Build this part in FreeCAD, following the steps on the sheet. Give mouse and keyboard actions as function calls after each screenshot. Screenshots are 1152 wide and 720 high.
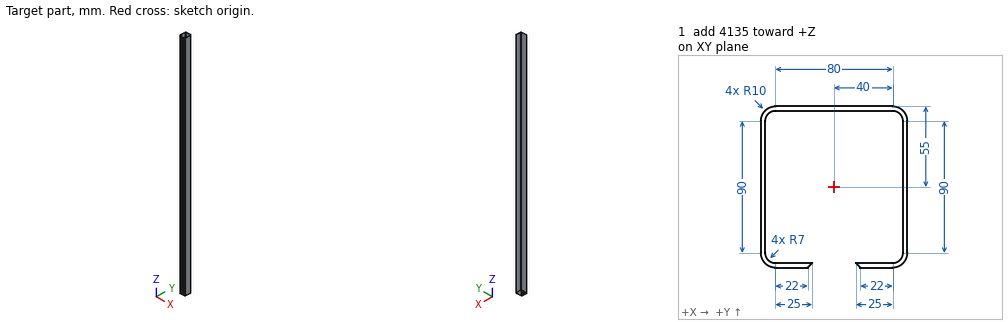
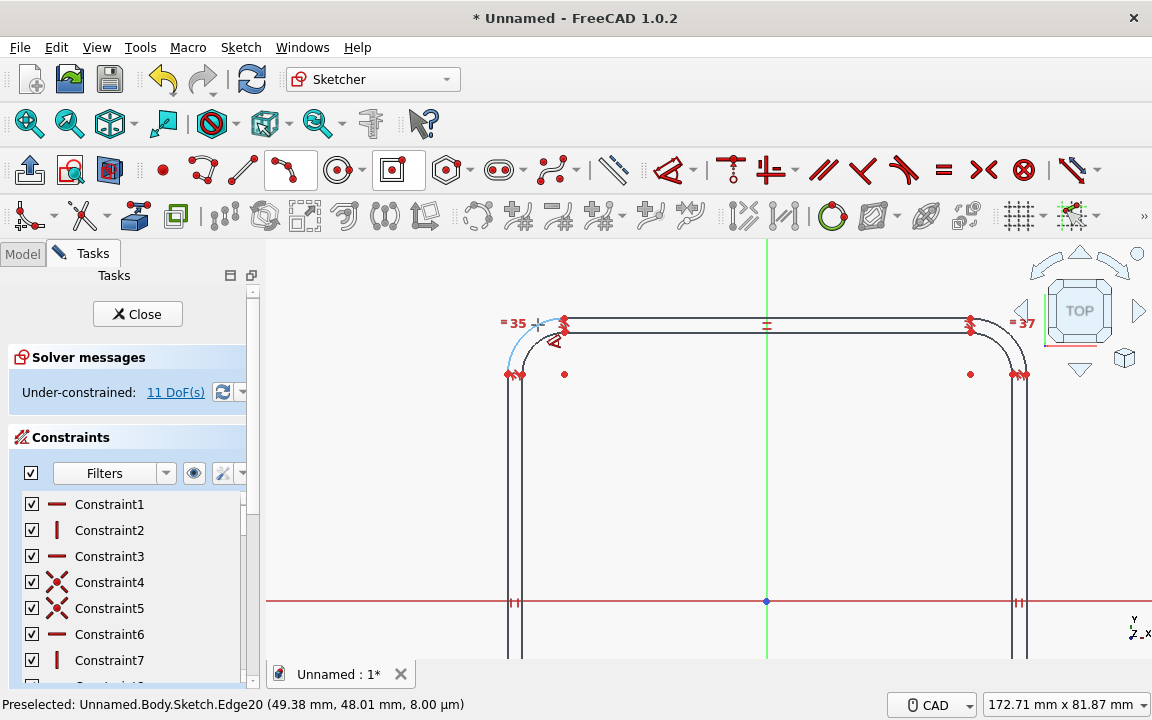
click(539, 325)
click(525, 296)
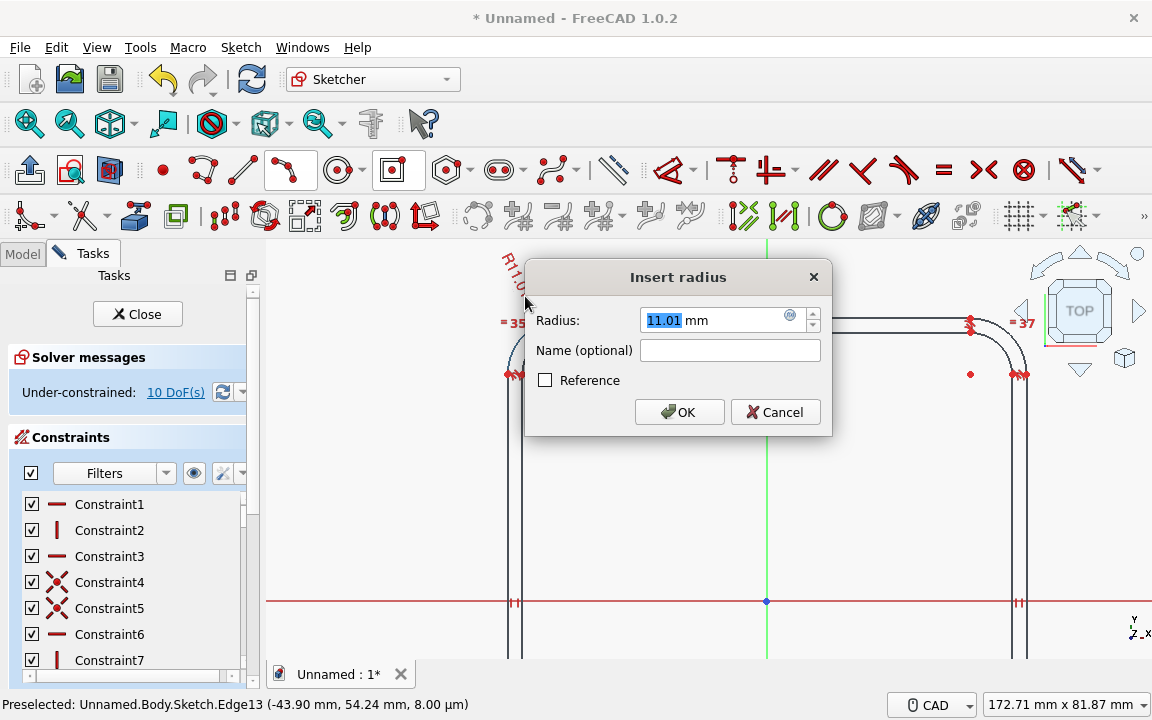
text(10)
key(Return)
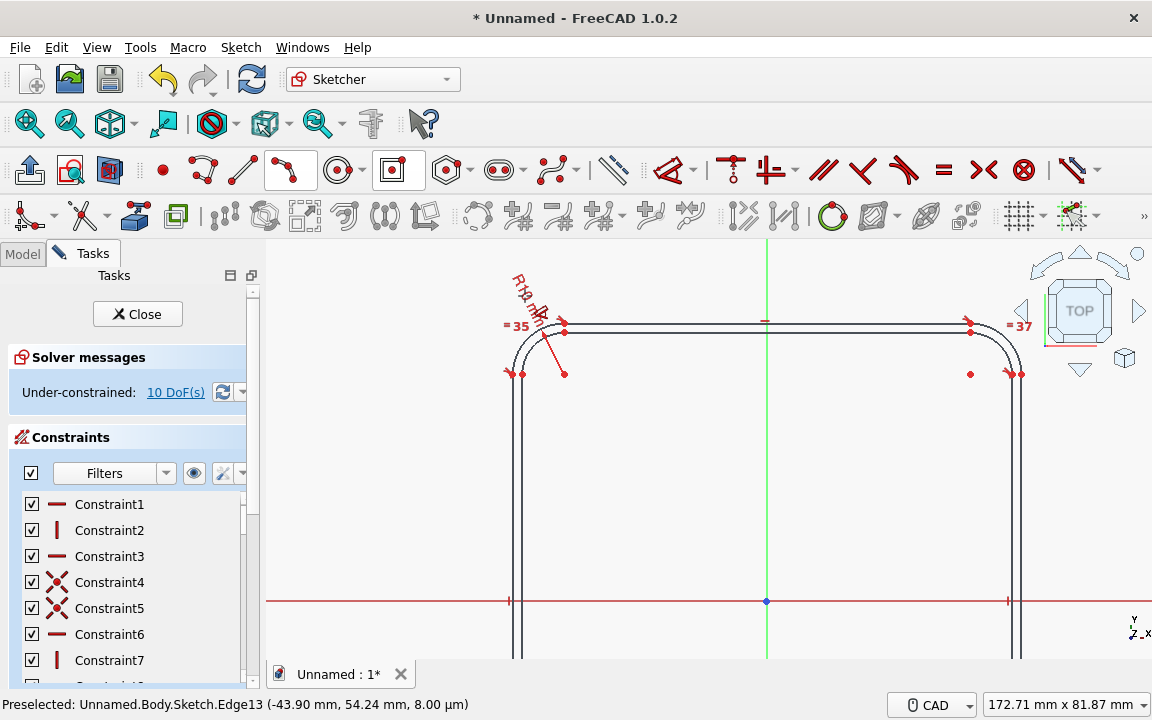
scroll(537, 325, down, 4)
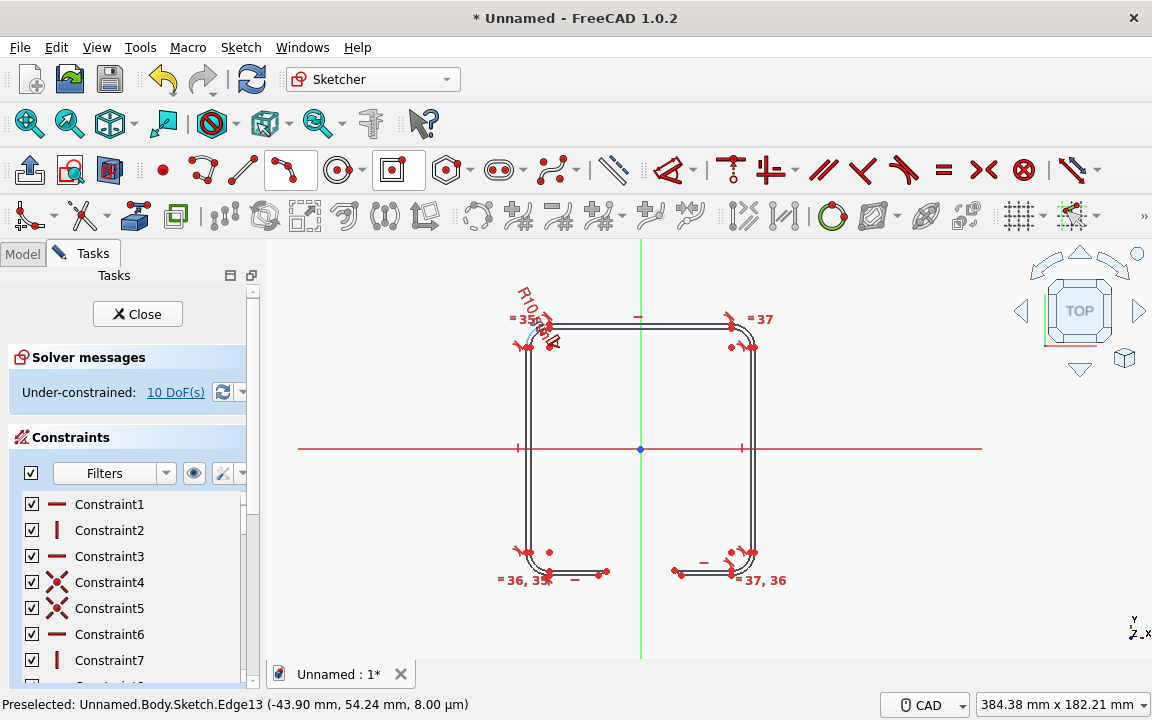
scroll(533, 561, up, 6)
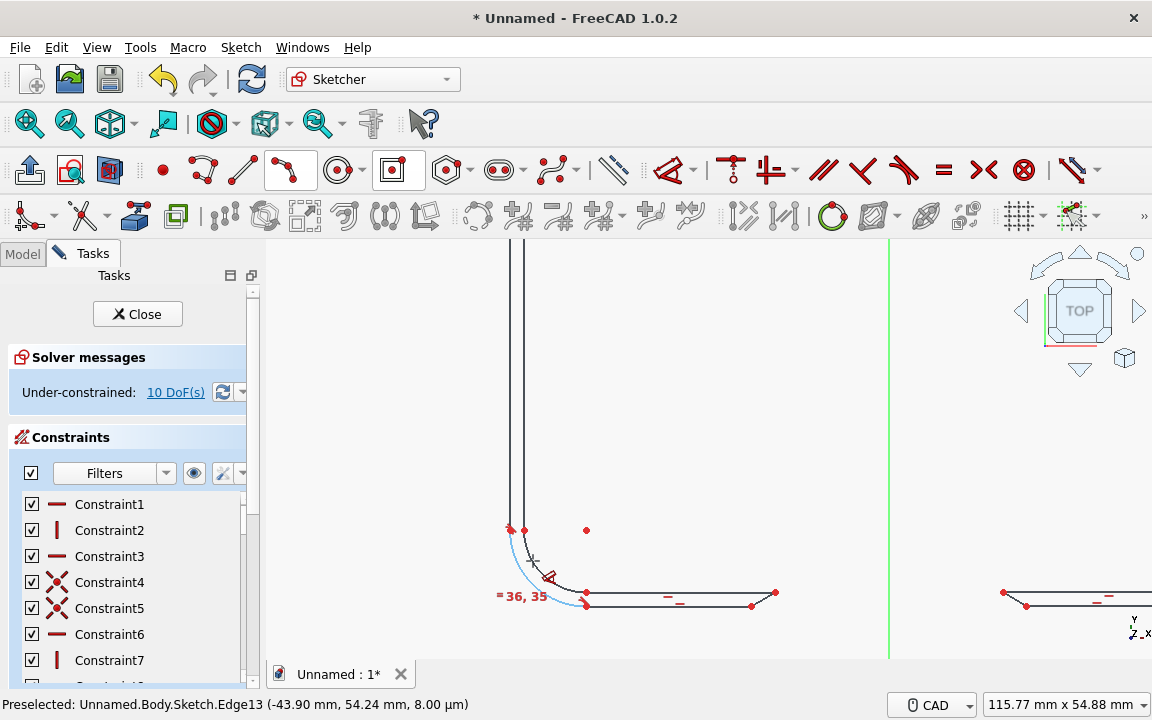
click(531, 558)
click(502, 572)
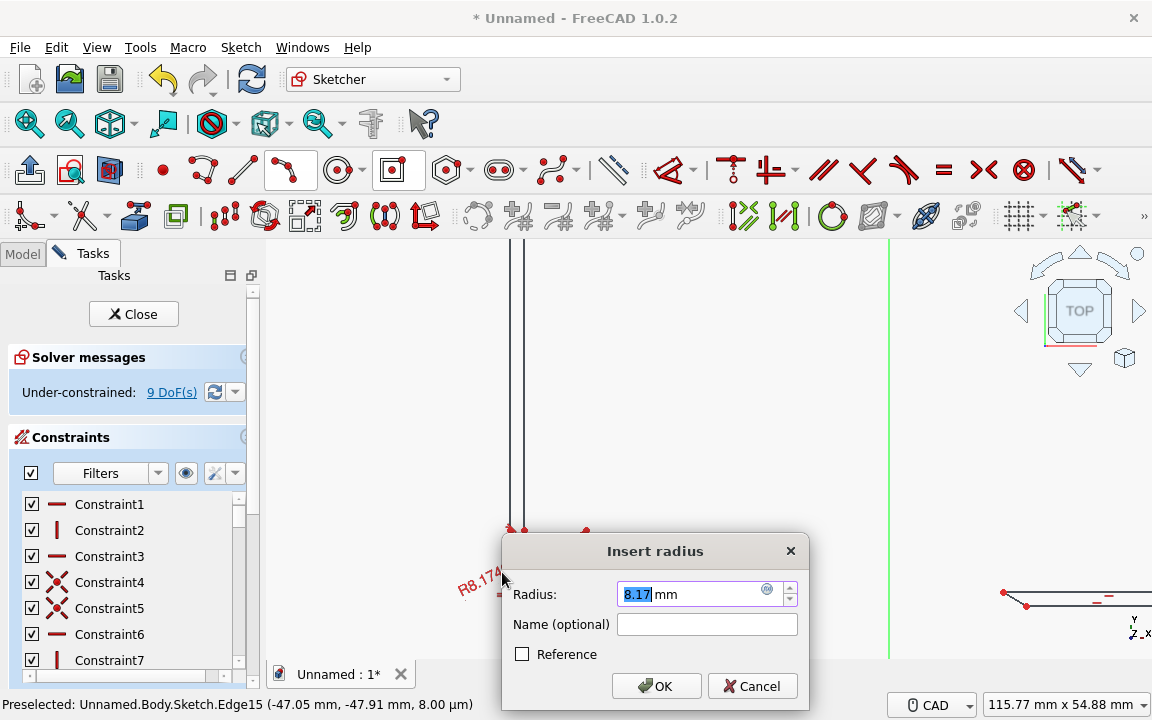
text(7)
key(Return)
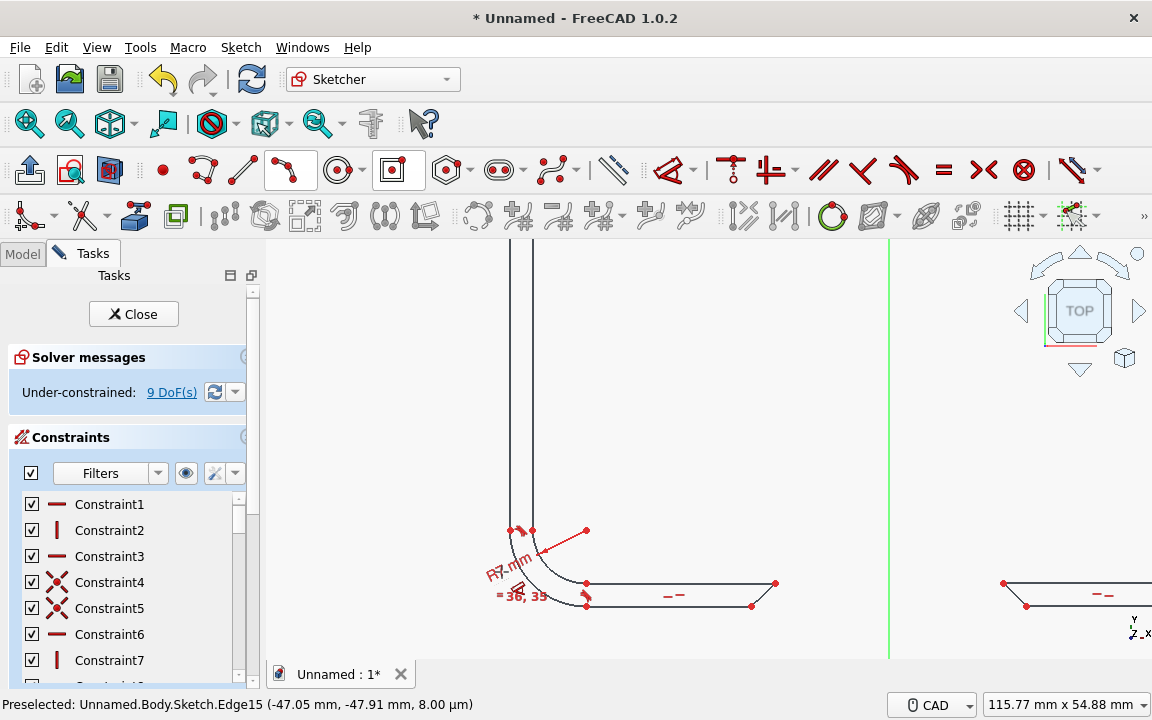
scroll(533, 561, down, 6)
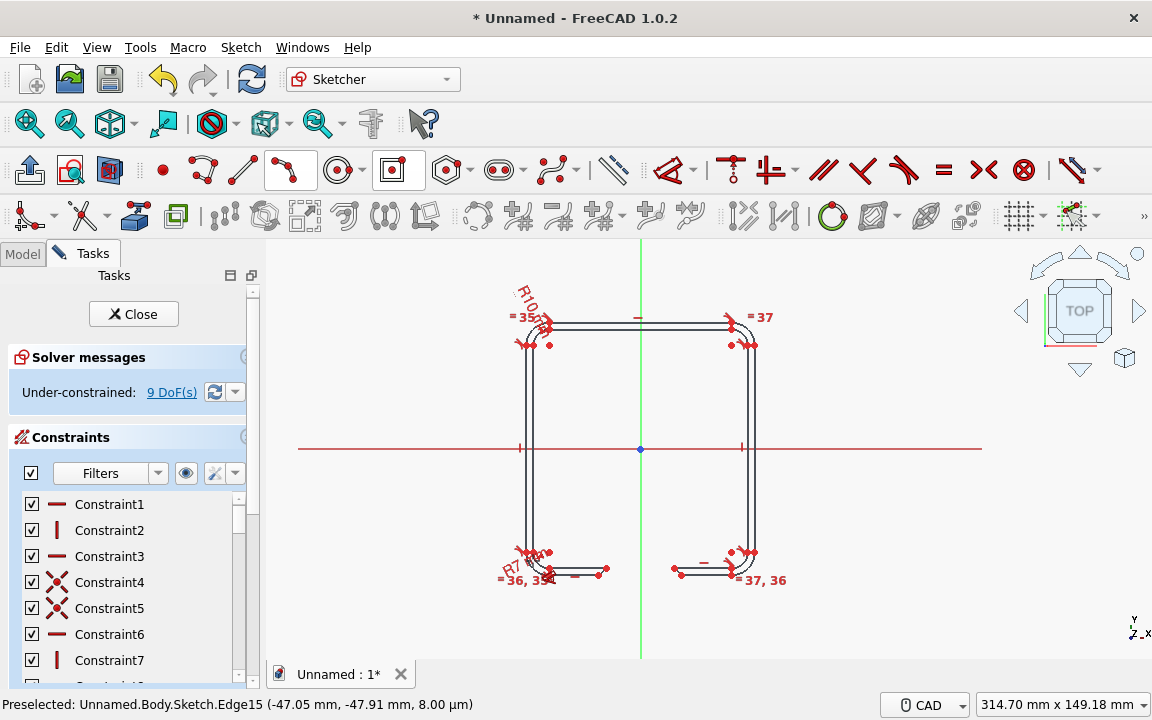
scroll(677, 323, up, 4)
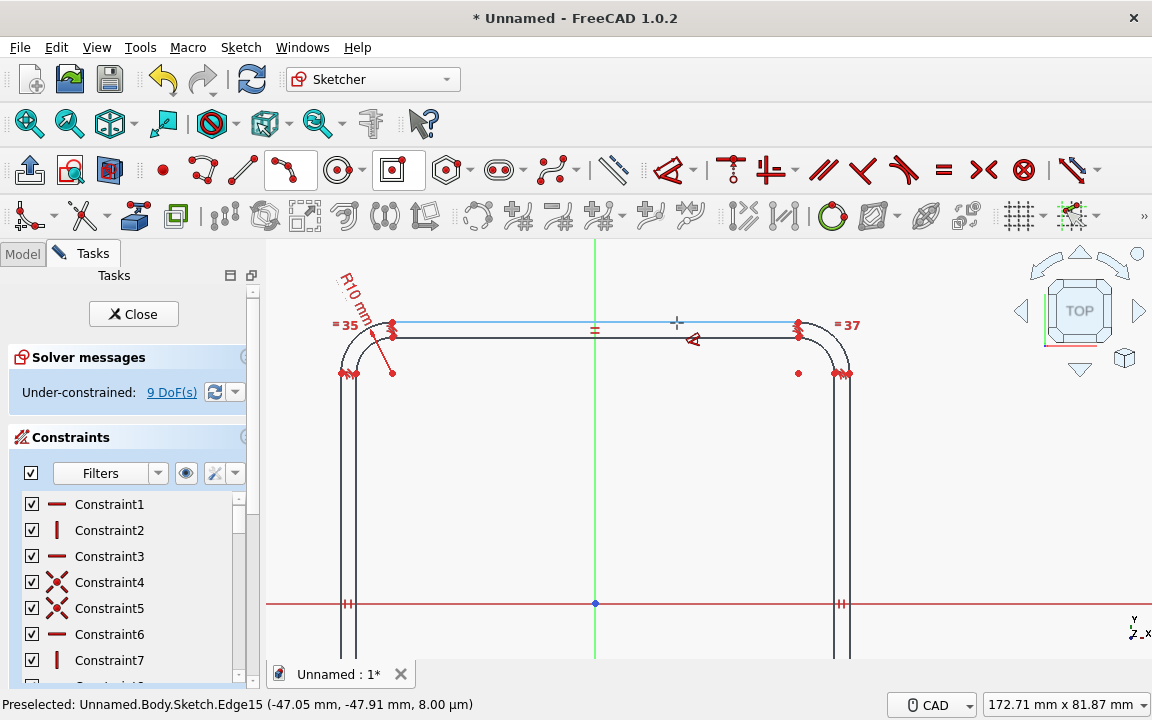
click(677, 322)
click(502, 288)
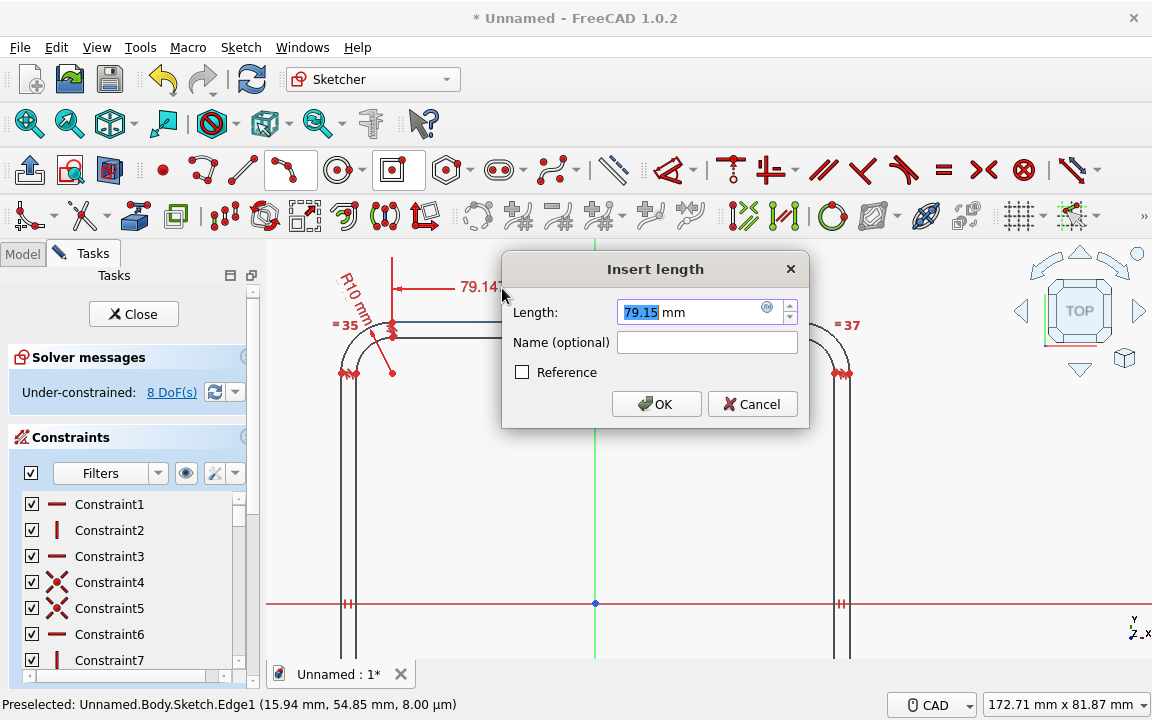
text(80)
key(Return)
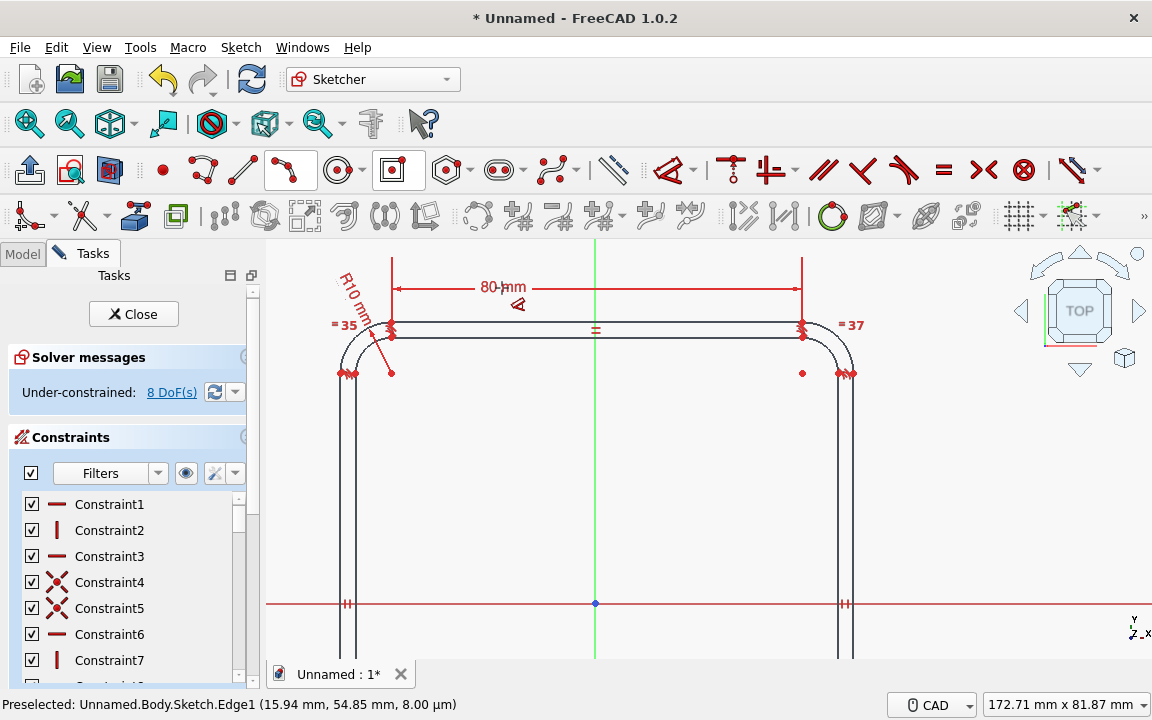
click(340, 511)
click(306, 502)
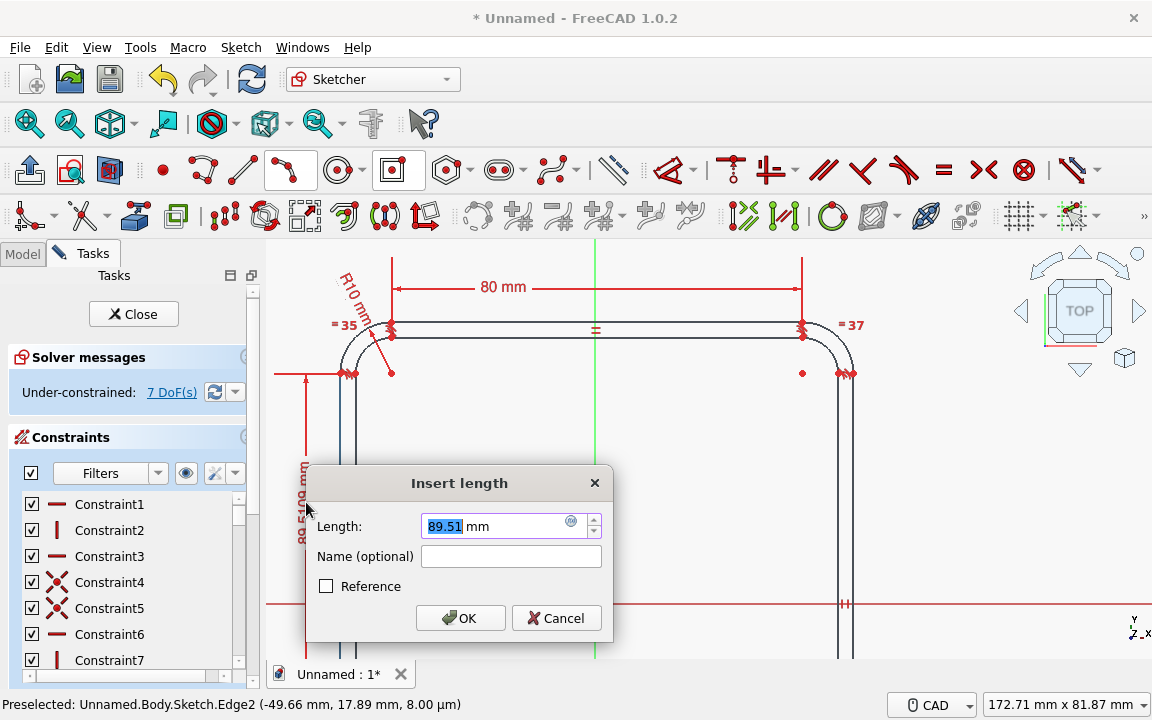
text(90)
key(Return)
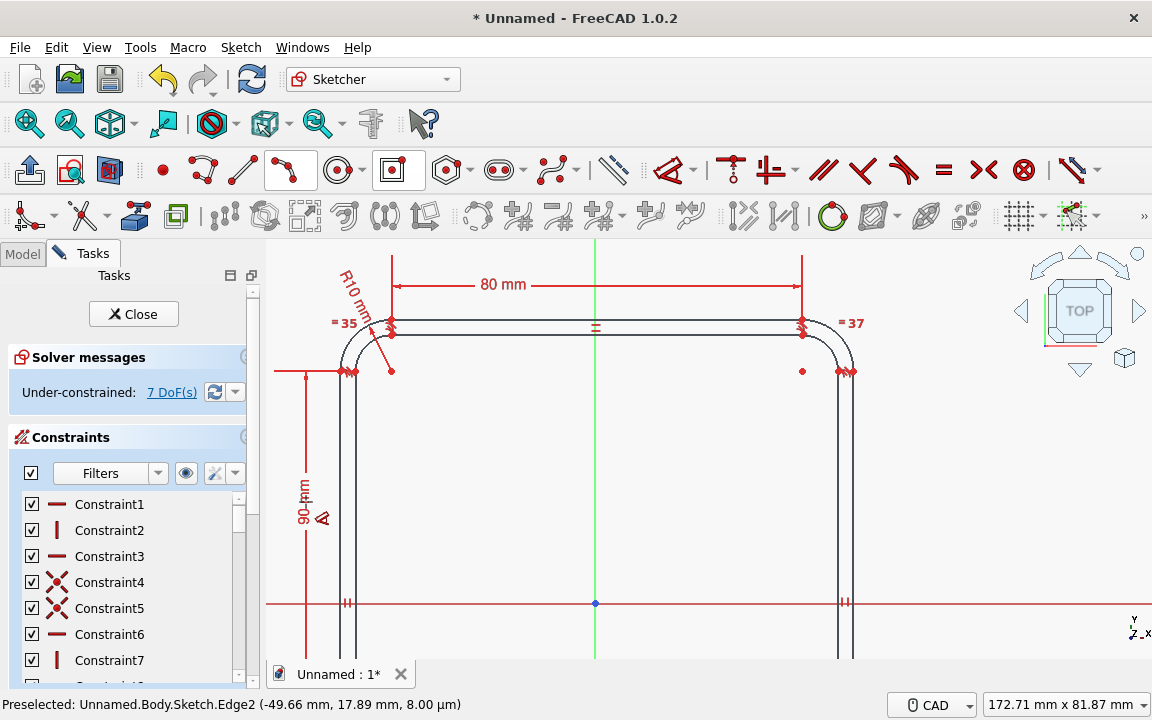
scroll(677, 323, down, 4)